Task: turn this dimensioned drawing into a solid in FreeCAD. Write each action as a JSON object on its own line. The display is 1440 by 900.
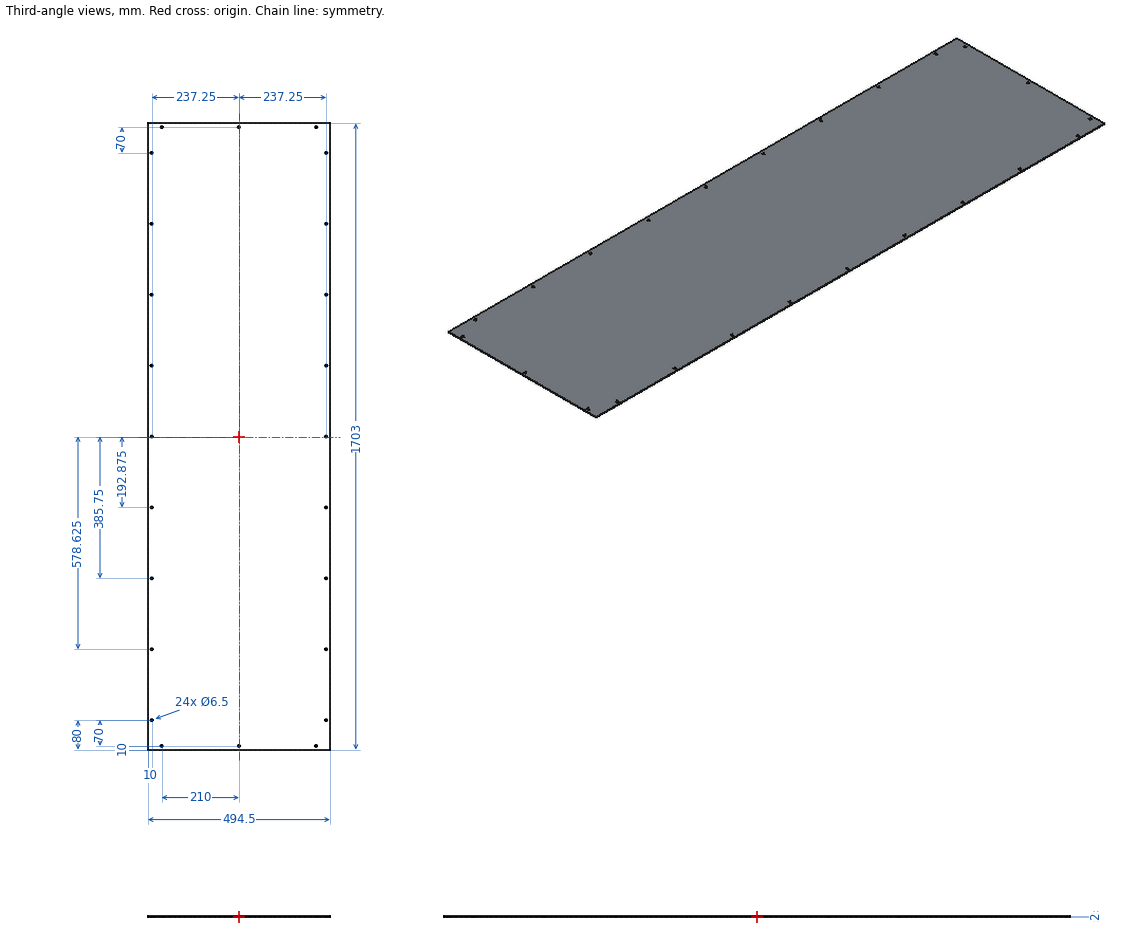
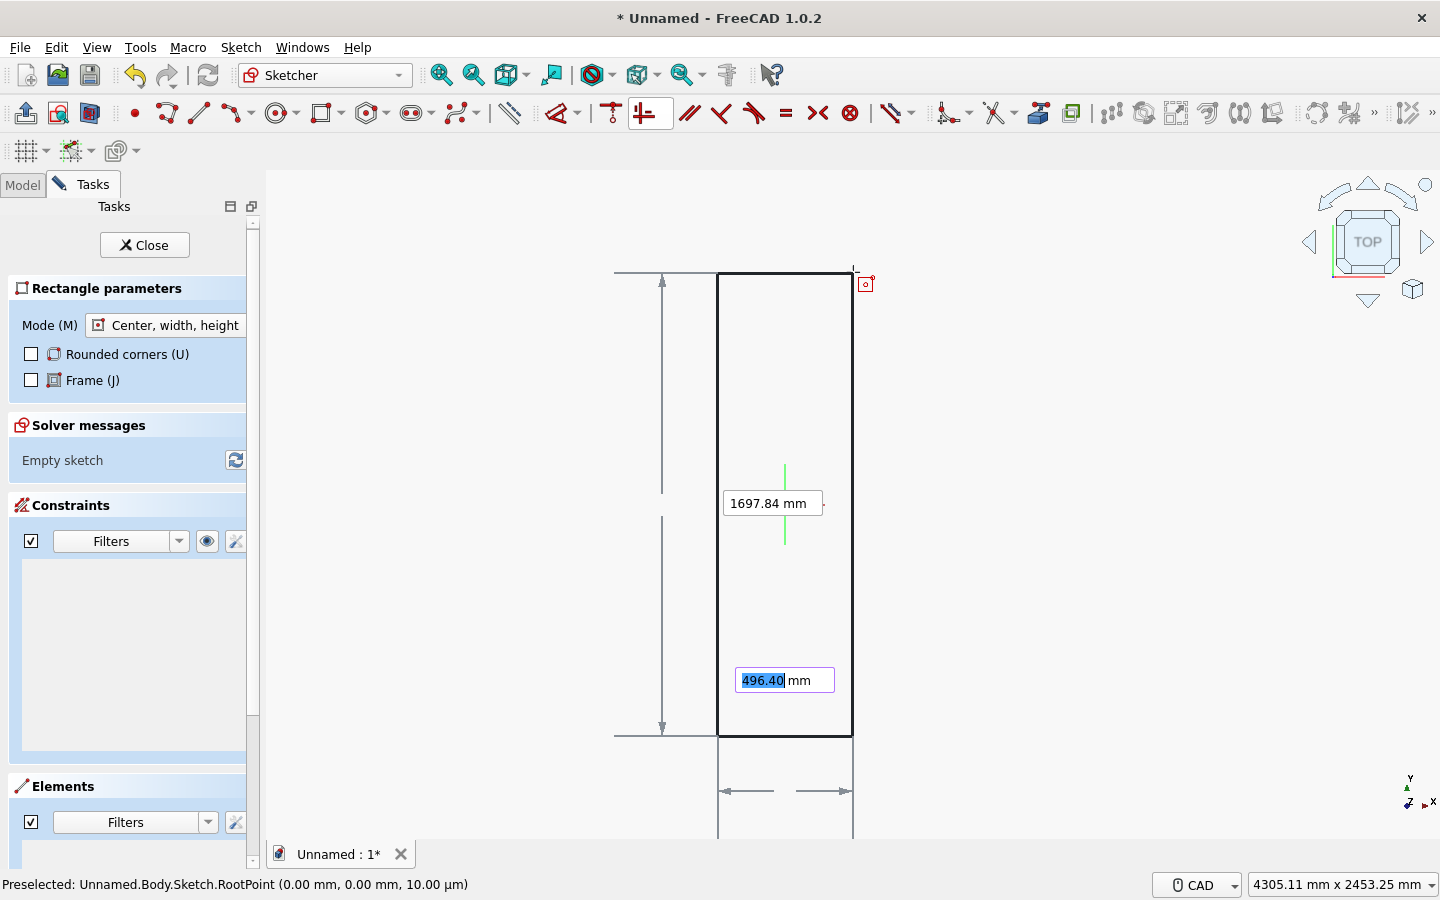
{"action": "type", "text": "494.5"}
{"action": "key", "text": "Tab"}
{"action": "type", "text": "1703"}
{"action": "key", "text": "Return"}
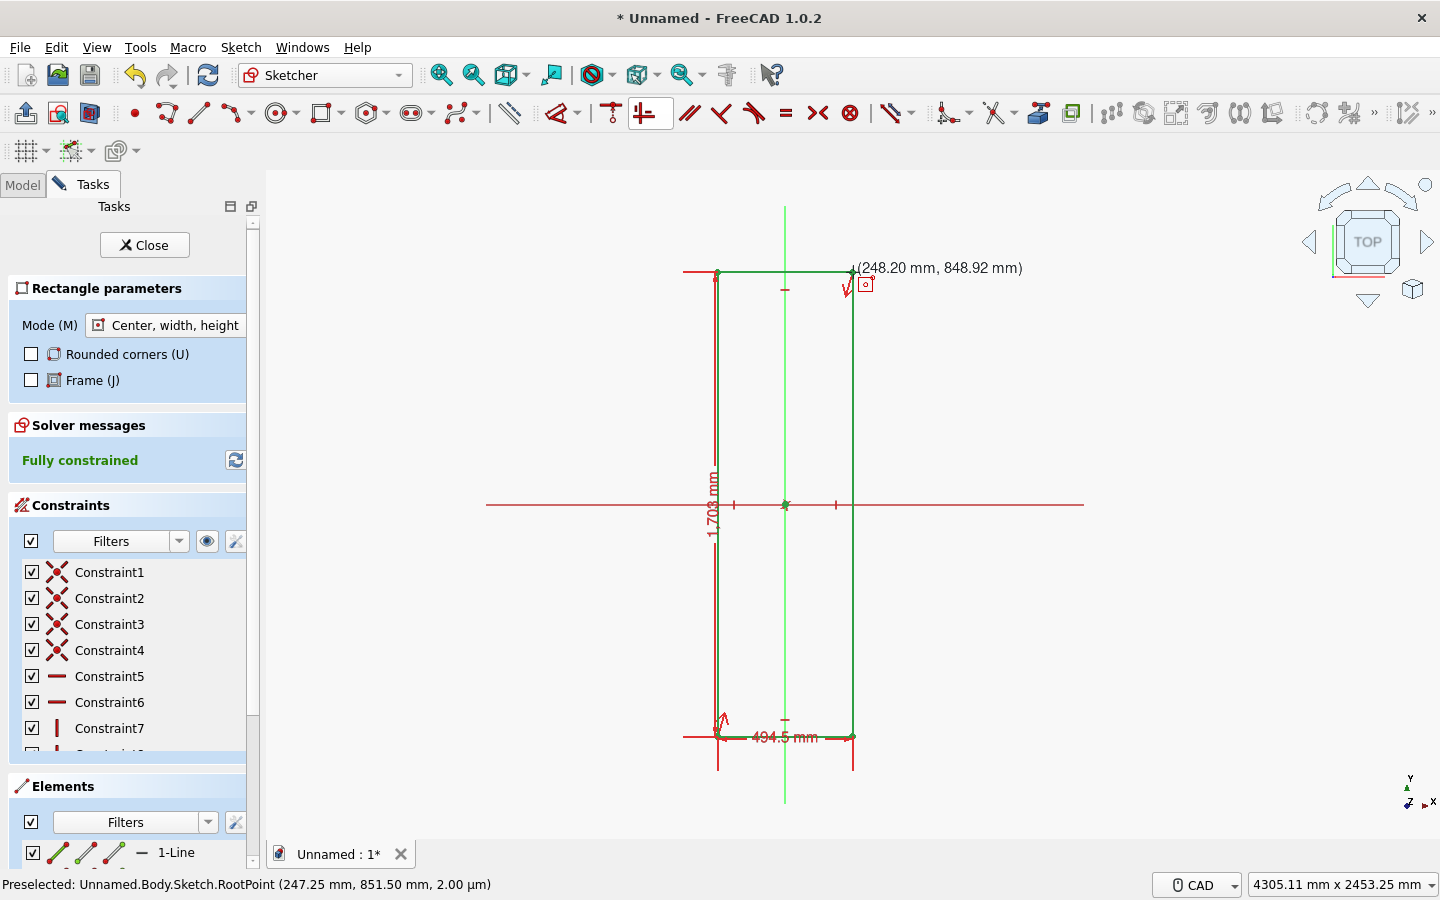
{"action": "left_click", "coordinate": [276, 114]}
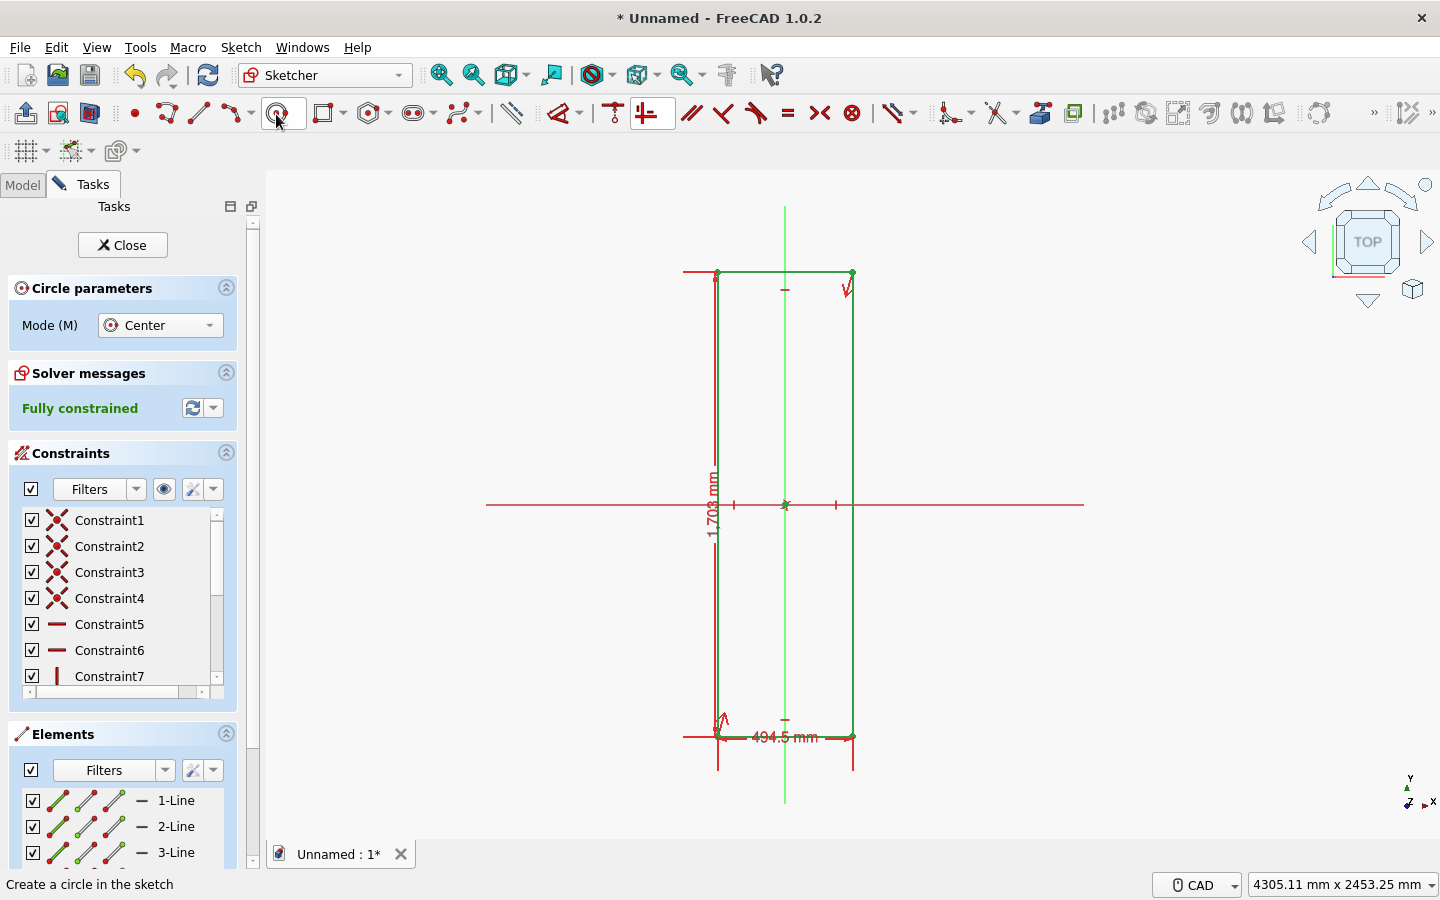
{"action": "scroll", "coordinate": [721, 715], "scroll_direction": "up", "scroll_amount": 17}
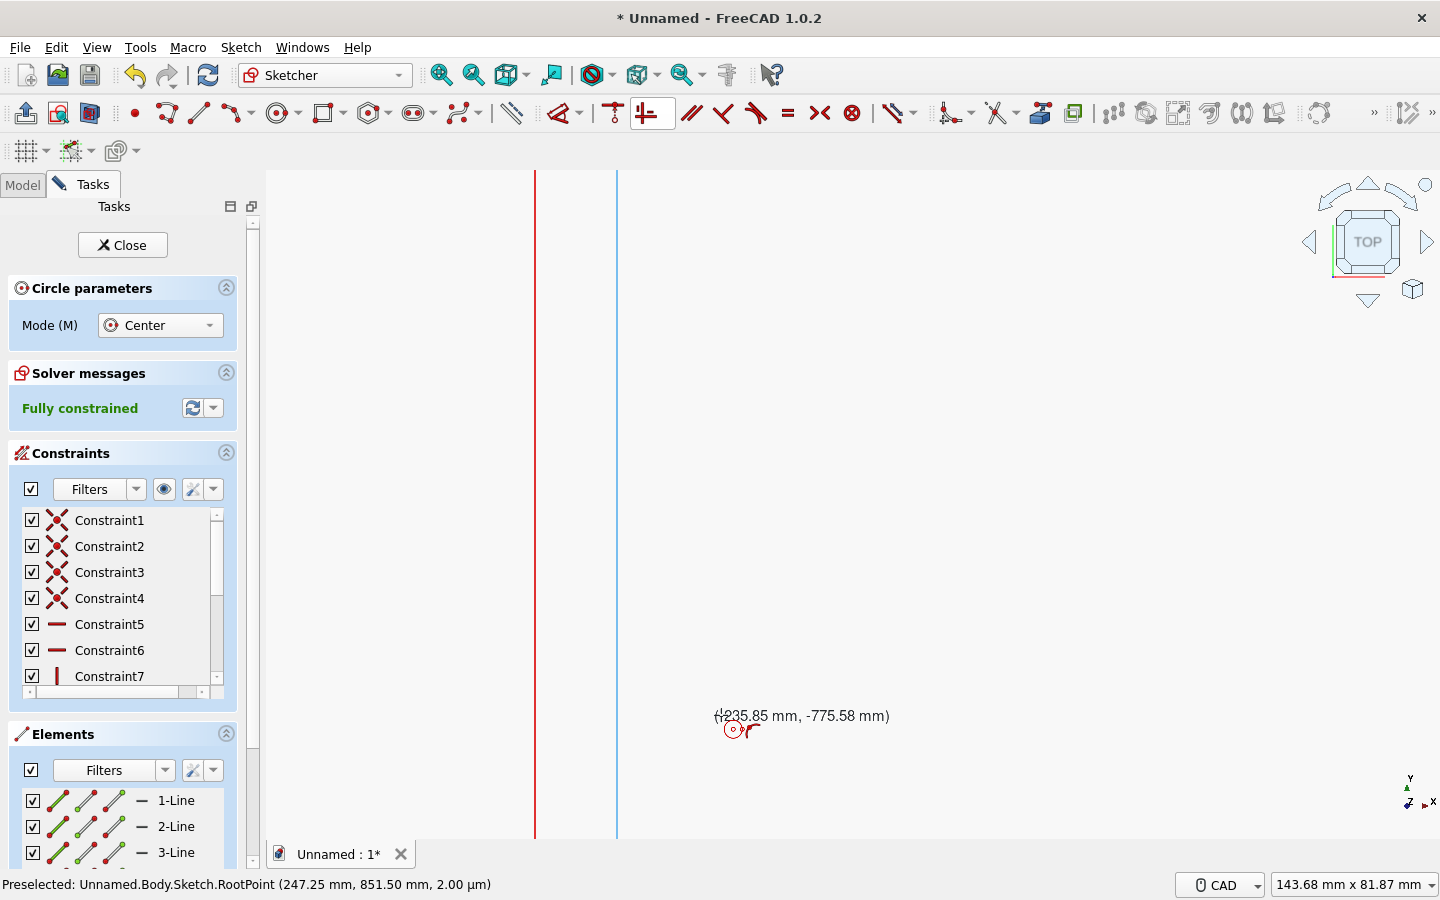
{"action": "scroll", "coordinate": [721, 716], "scroll_direction": "down", "scroll_amount": 17}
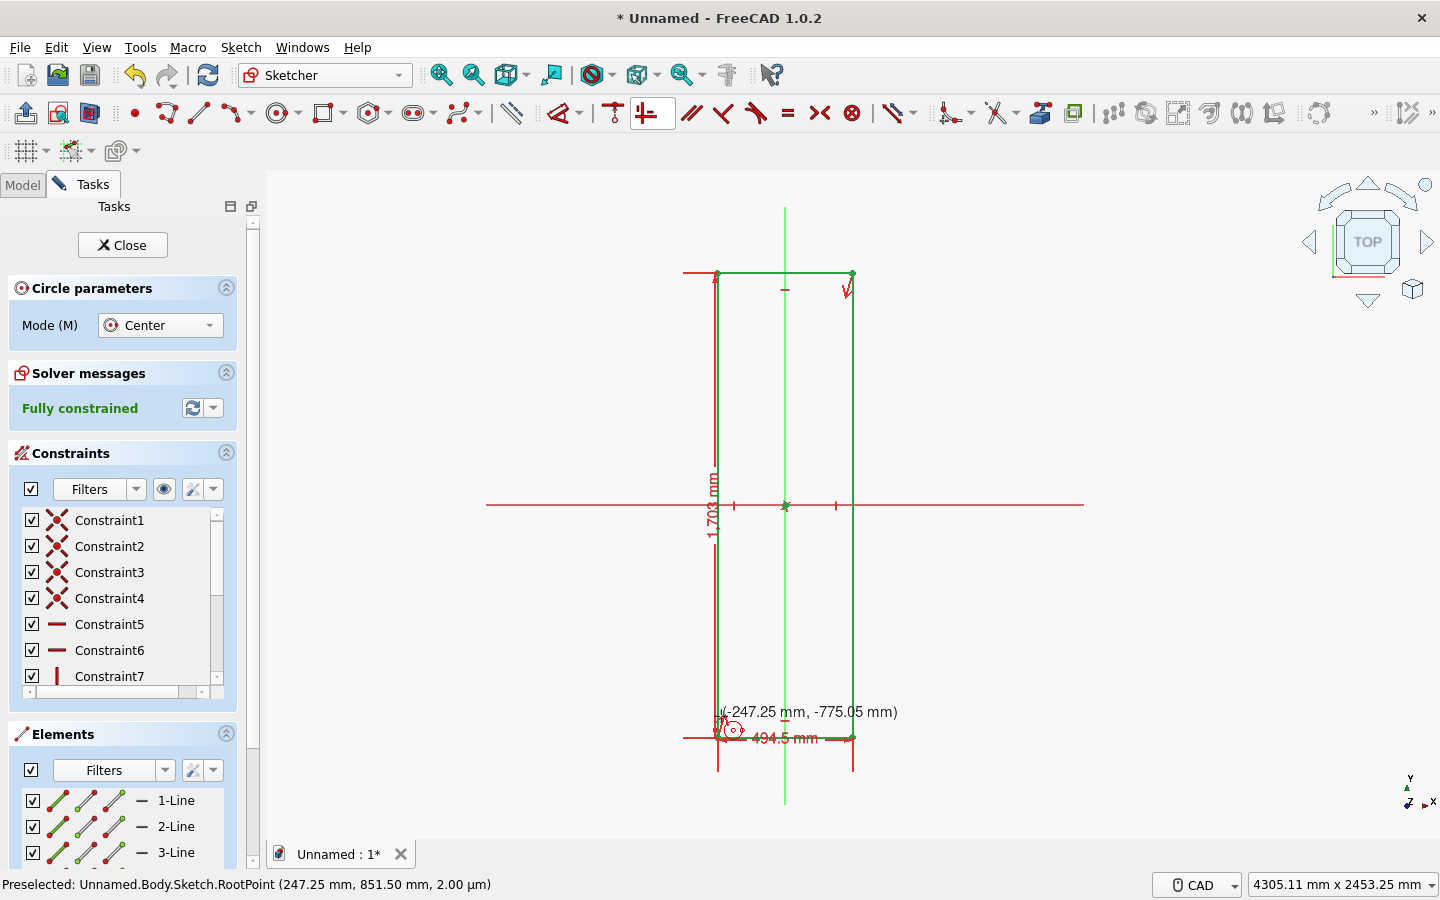
{"action": "scroll", "coordinate": [721, 716], "scroll_direction": "up", "scroll_amount": 9}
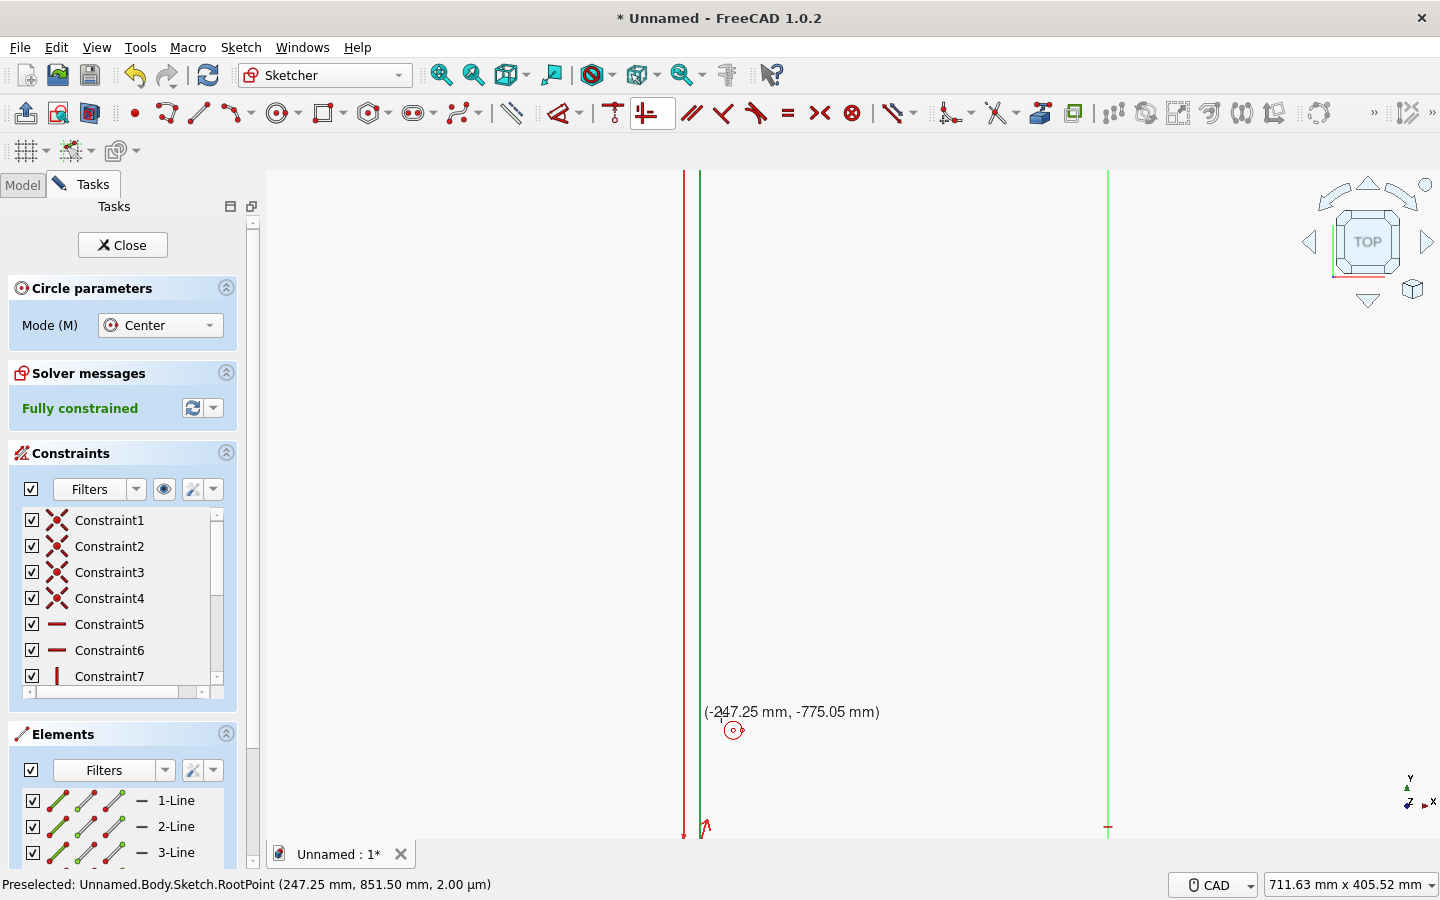
{"action": "left_click", "coordinate": [717, 711]}
{"action": "mouse_move", "coordinate": [721, 707]}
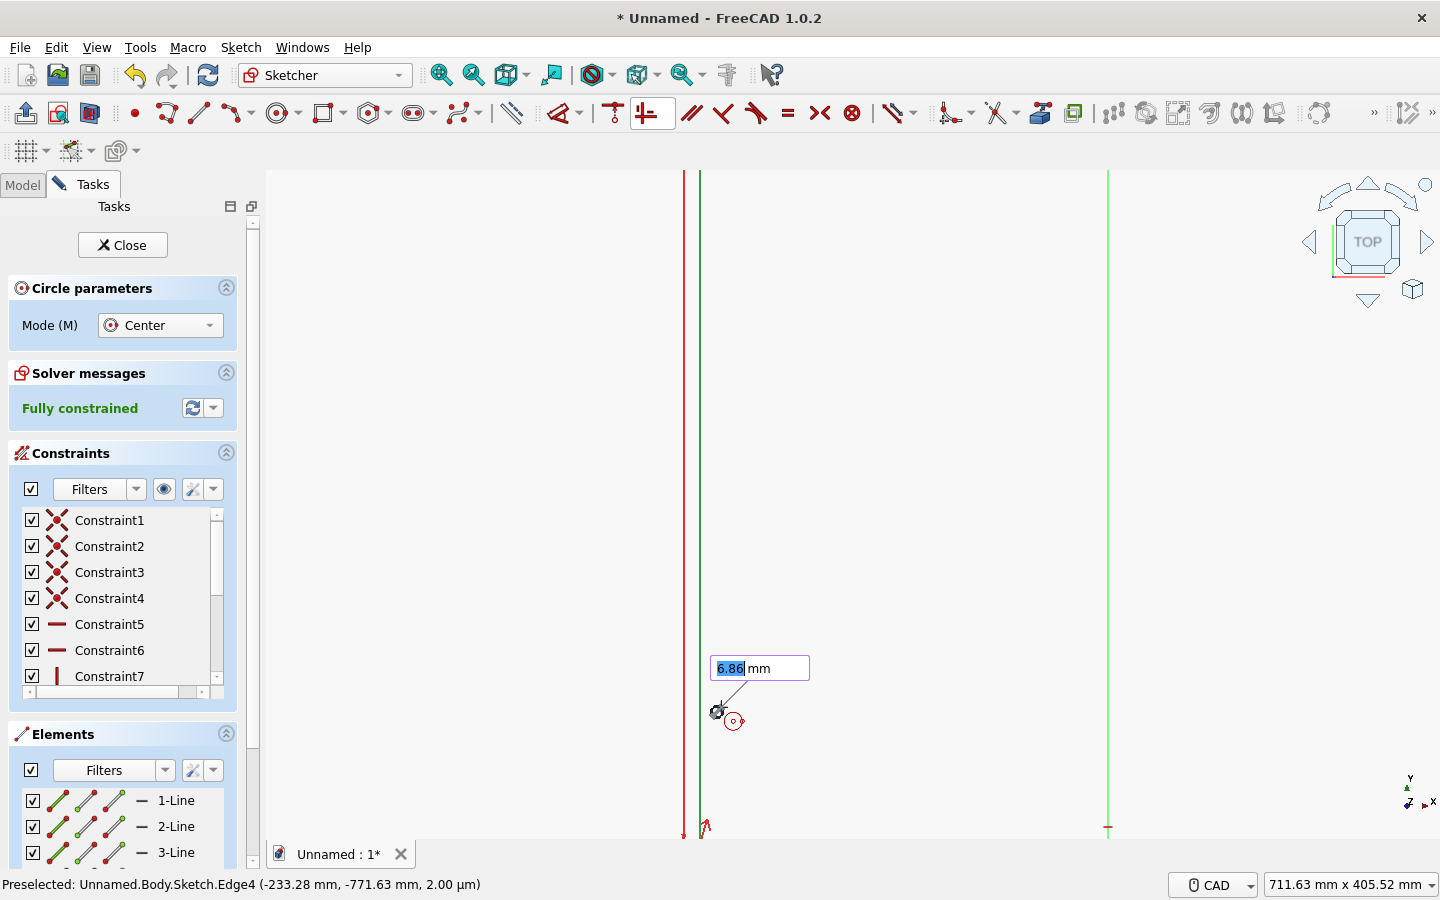
{"action": "type", "text": "6.5"}
{"action": "key", "text": "Return"}